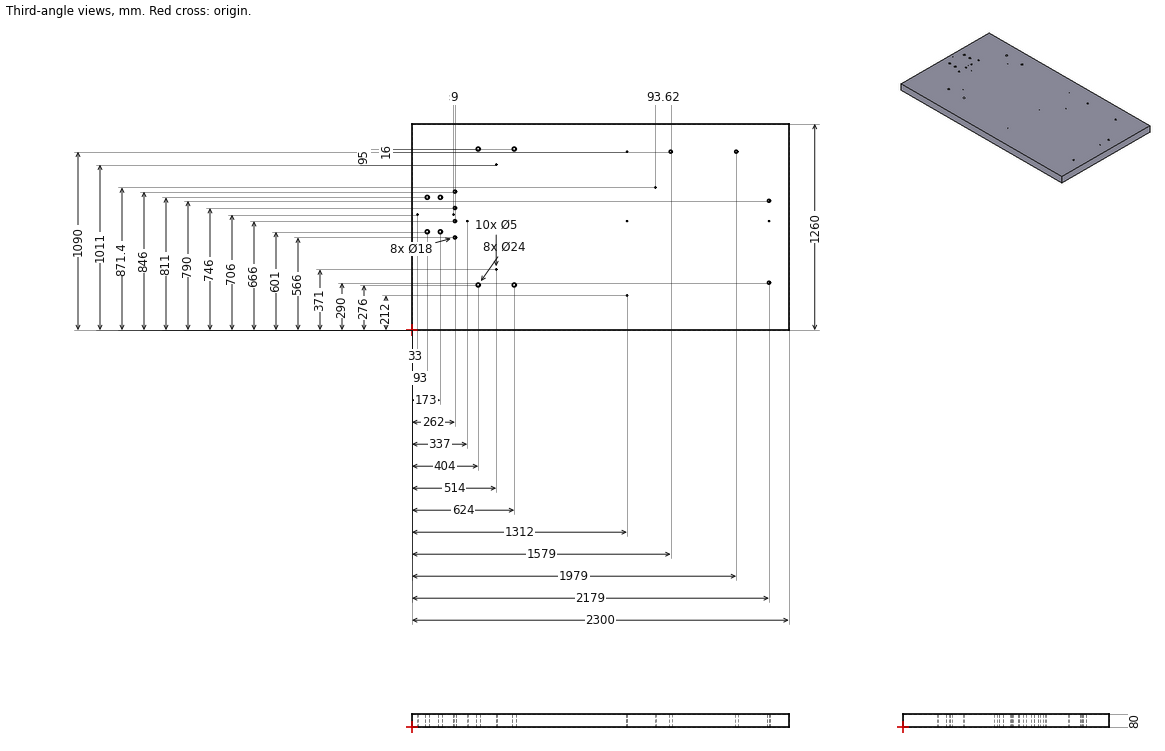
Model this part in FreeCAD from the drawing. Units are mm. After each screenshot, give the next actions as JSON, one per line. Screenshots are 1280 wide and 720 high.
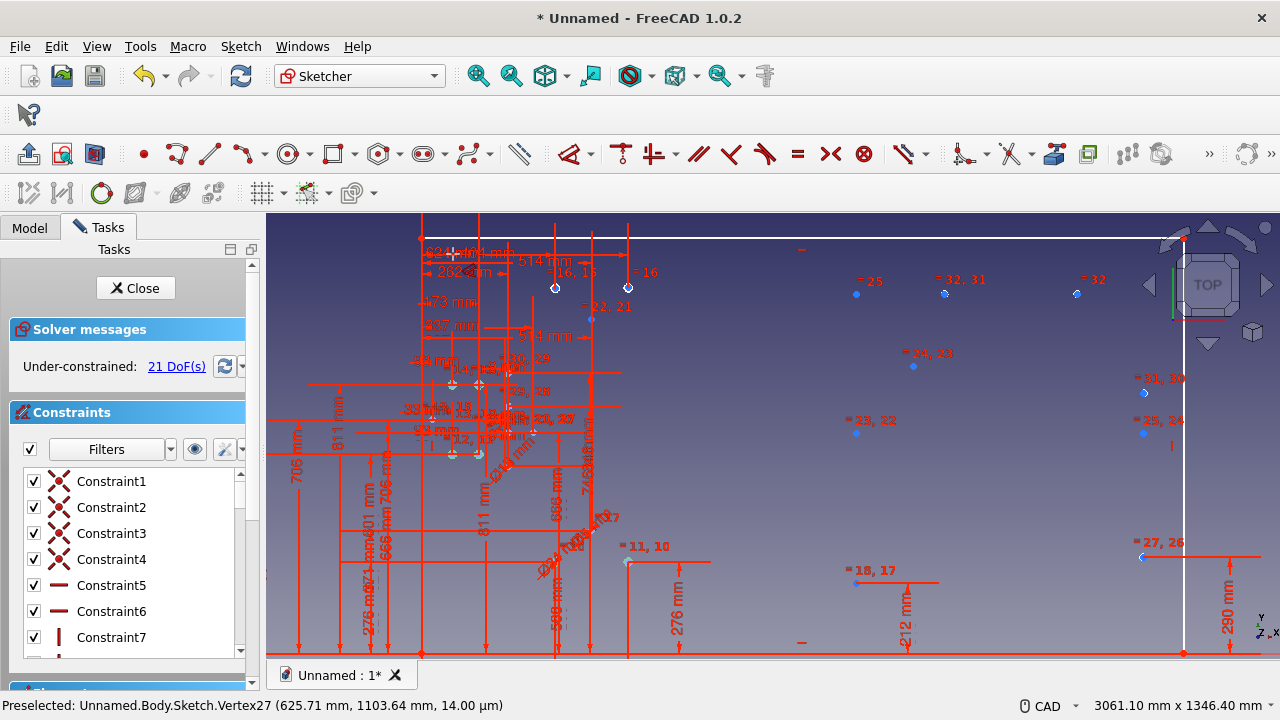
{"action": "left_click", "coordinate": [856, 434]}
{"action": "left_click", "coordinate": [890, 532]}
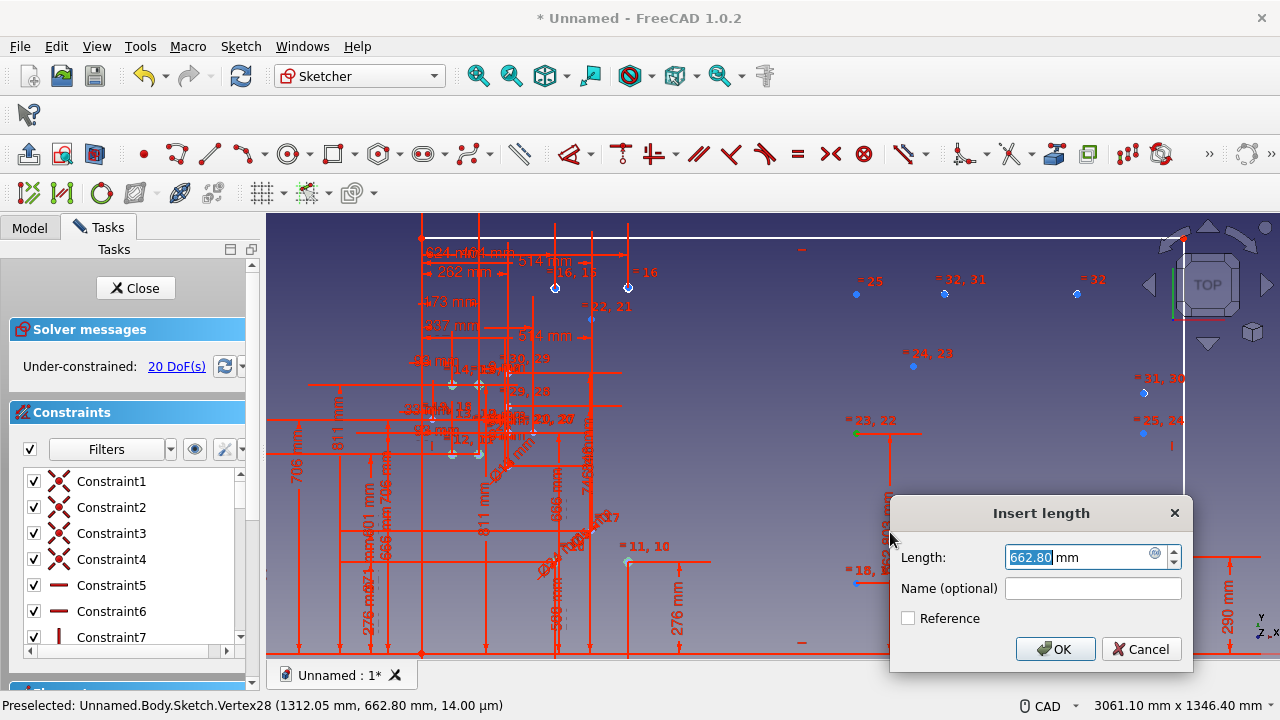
{"action": "type", "text": "666"}
{"action": "key", "text": "Return"}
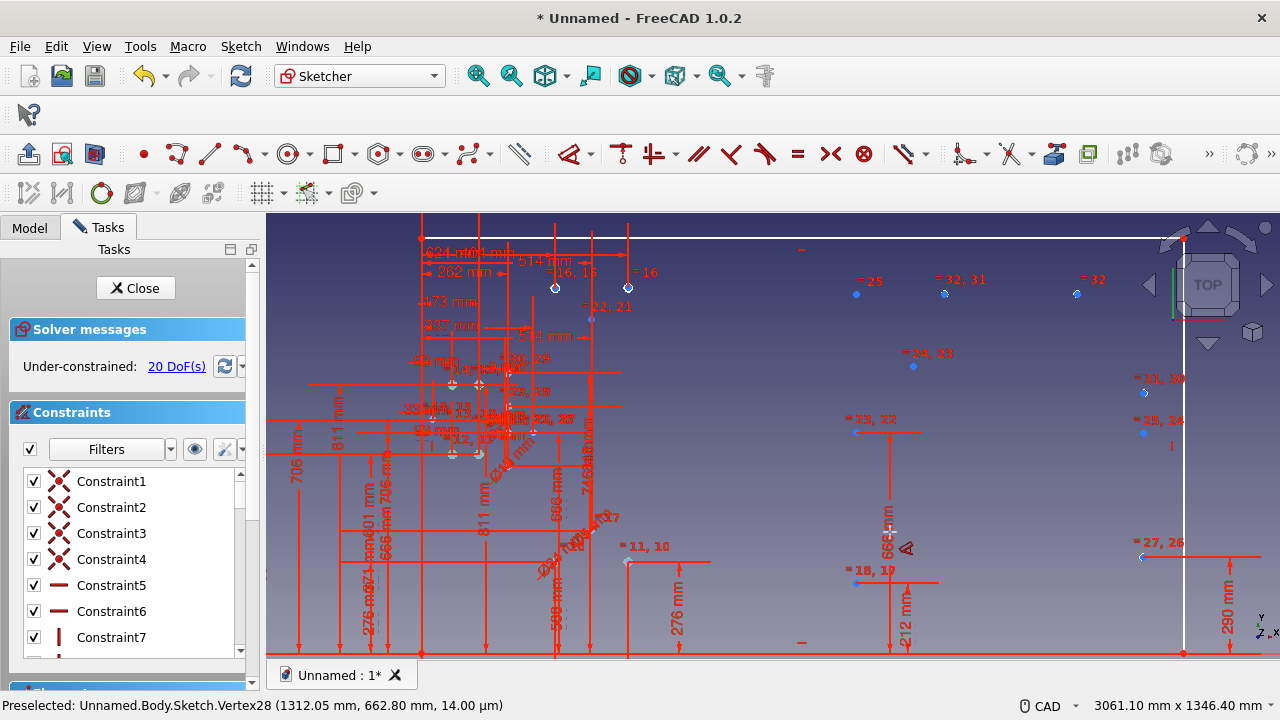
{"action": "scroll", "coordinate": [505, 418], "scroll_direction": "down", "scroll_amount": 2}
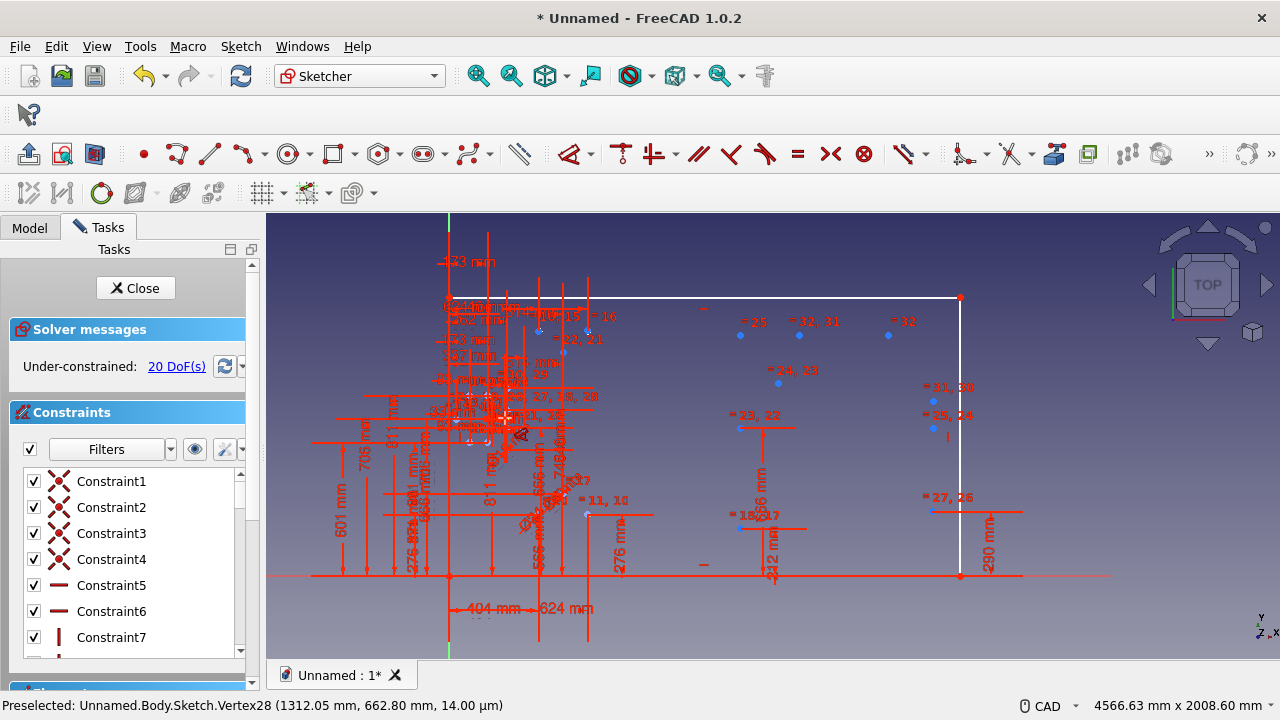
{"action": "left_click", "coordinate": [933, 429]}
{"action": "left_click", "coordinate": [991, 502]}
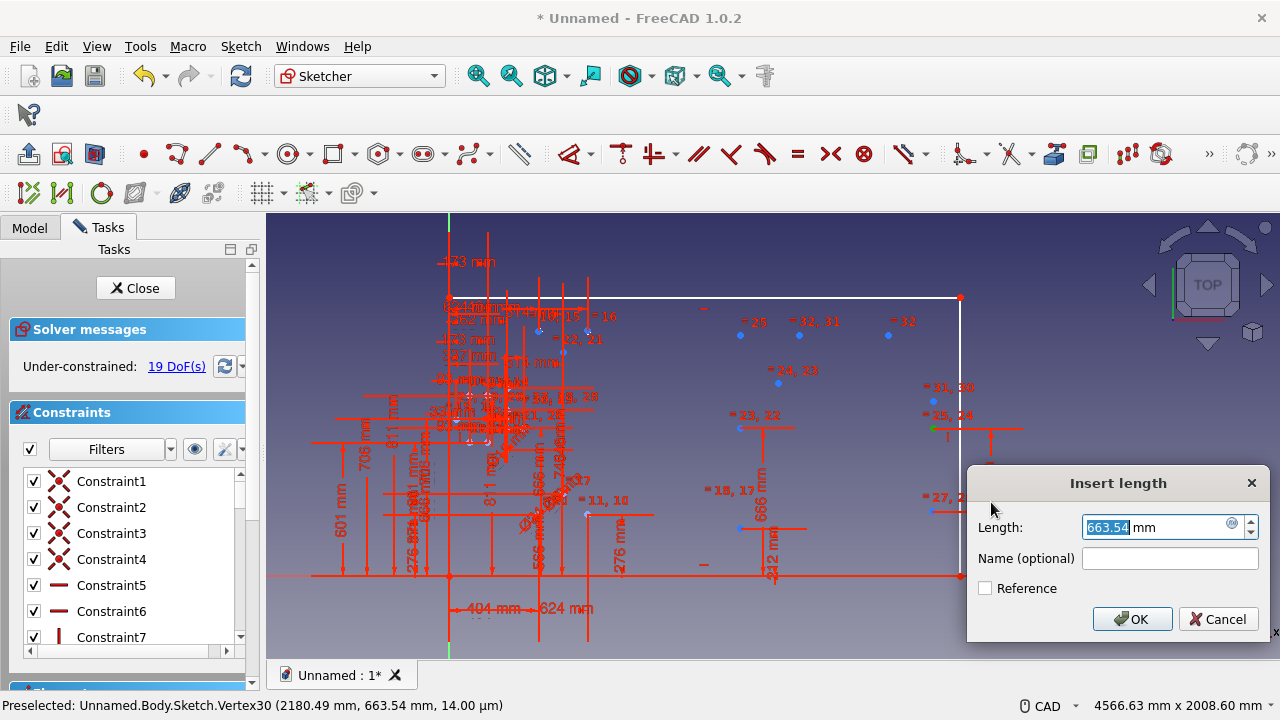
{"action": "type", "text": "666"}
{"action": "key", "text": "Return"}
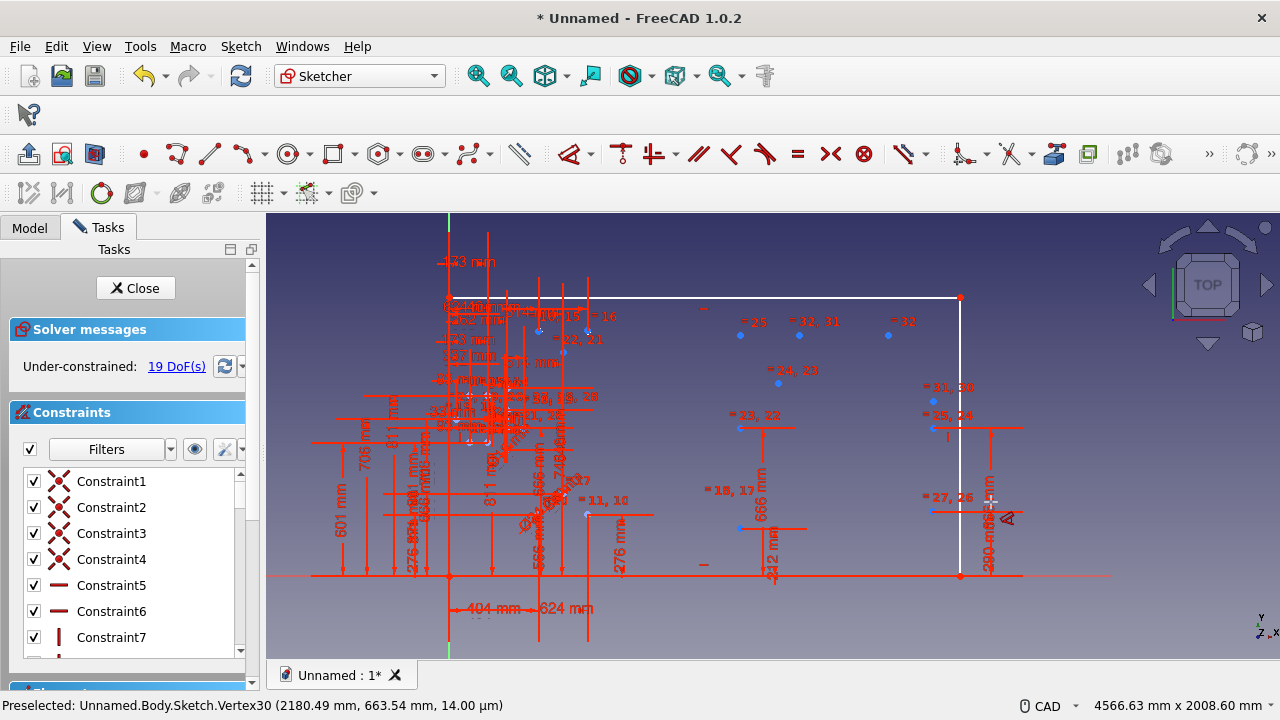
{"action": "left_click", "coordinate": [933, 402]}
{"action": "left_click", "coordinate": [991, 449]}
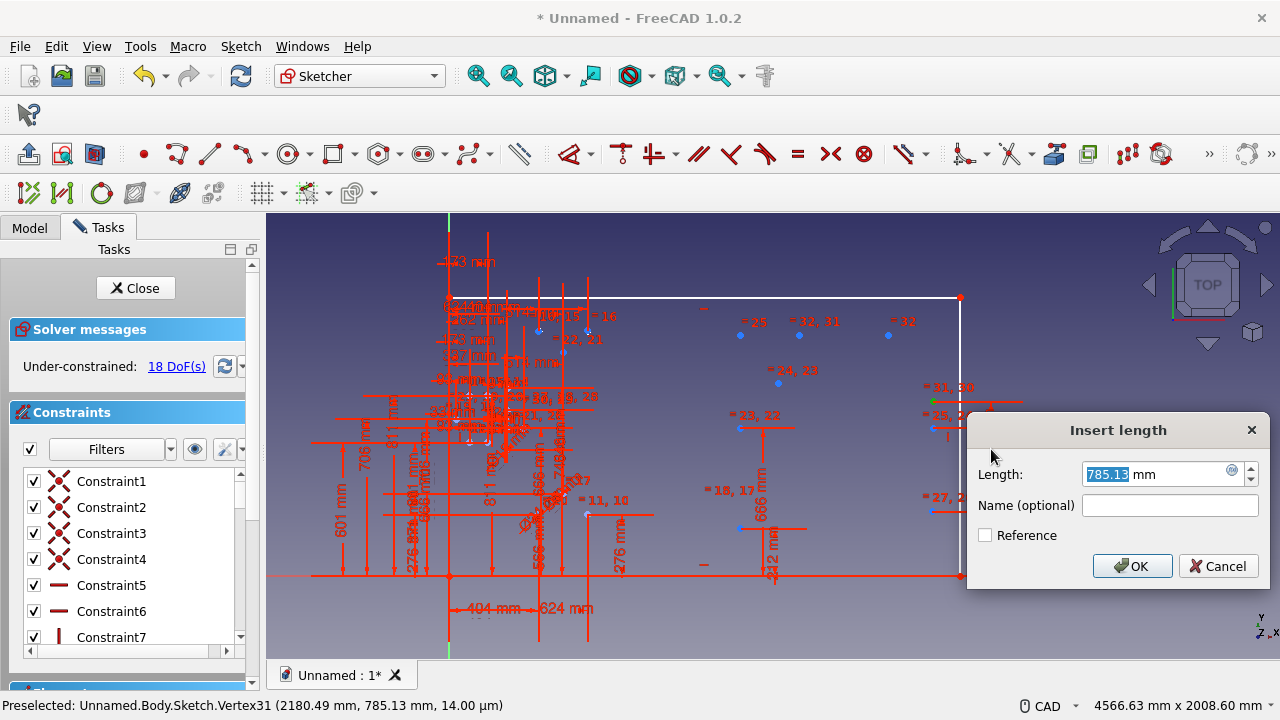
{"action": "type", "text": "790"}
{"action": "key", "text": "Return"}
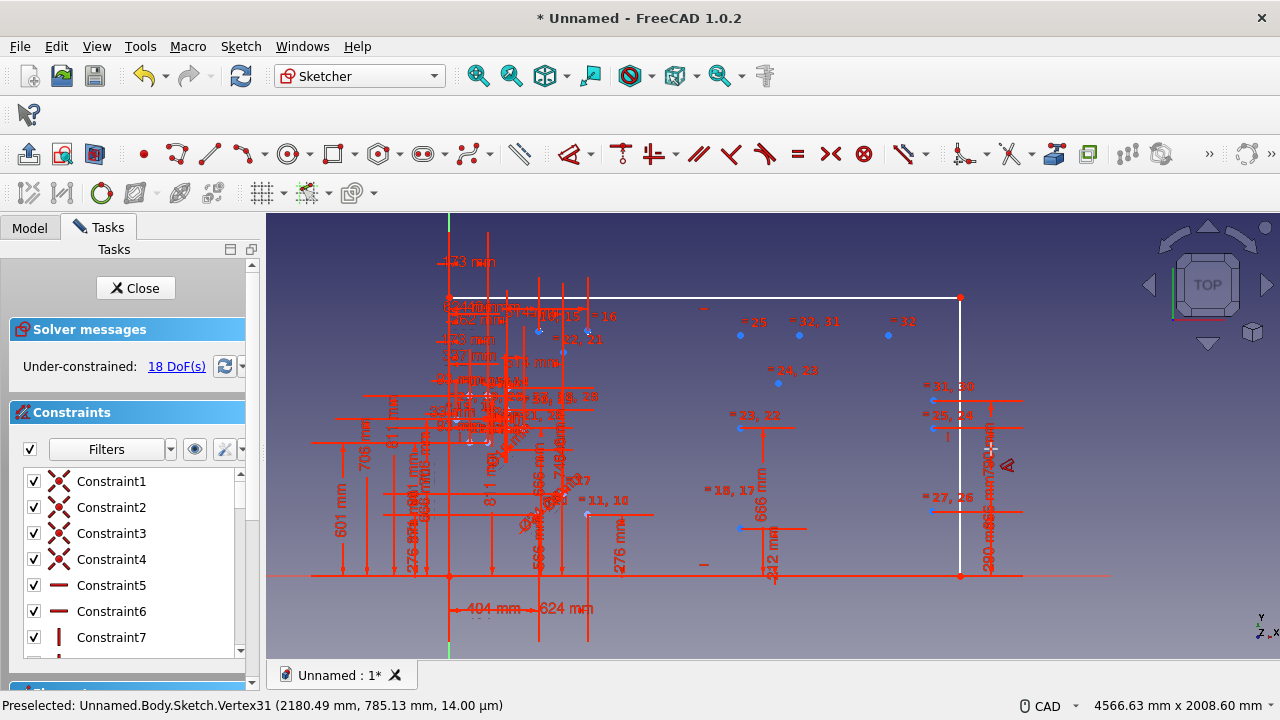
{"action": "scroll", "coordinate": [563, 352], "scroll_direction": "up", "scroll_amount": 4}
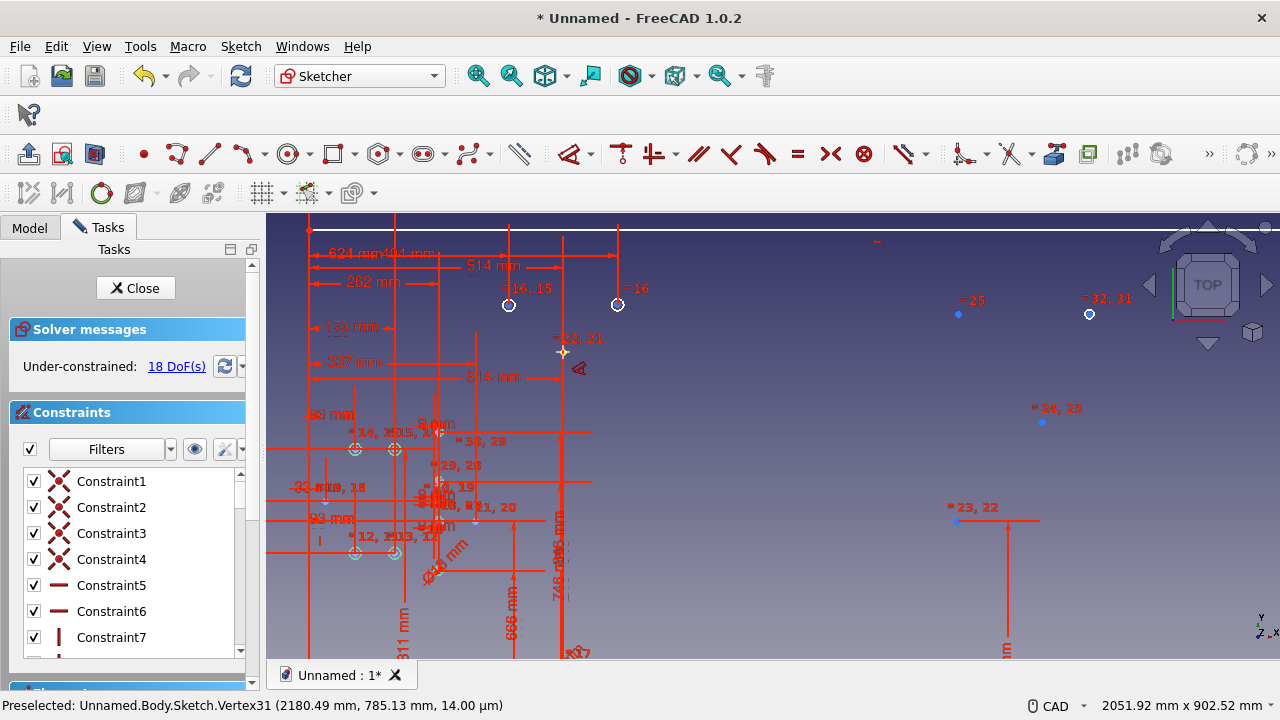
{"action": "left_click", "coordinate": [563, 352]}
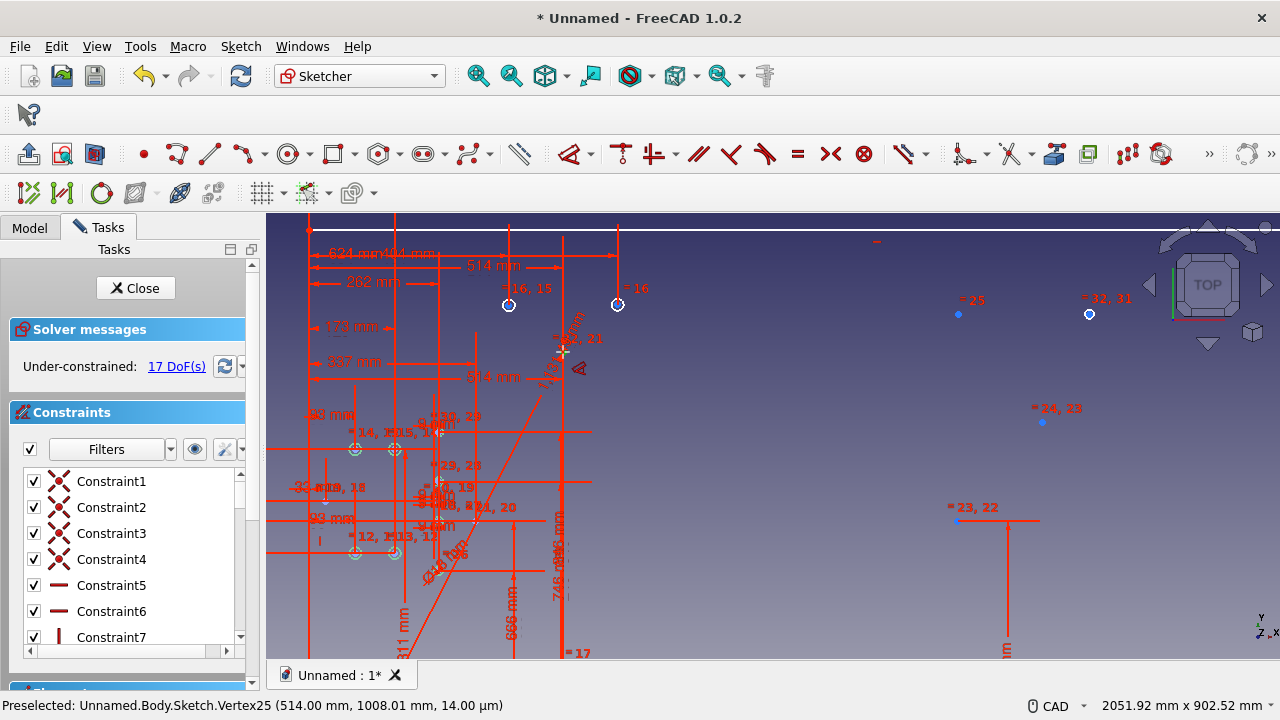
{"action": "left_click", "coordinate": [509, 305]}
{"action": "left_click", "coordinate": [475, 329]}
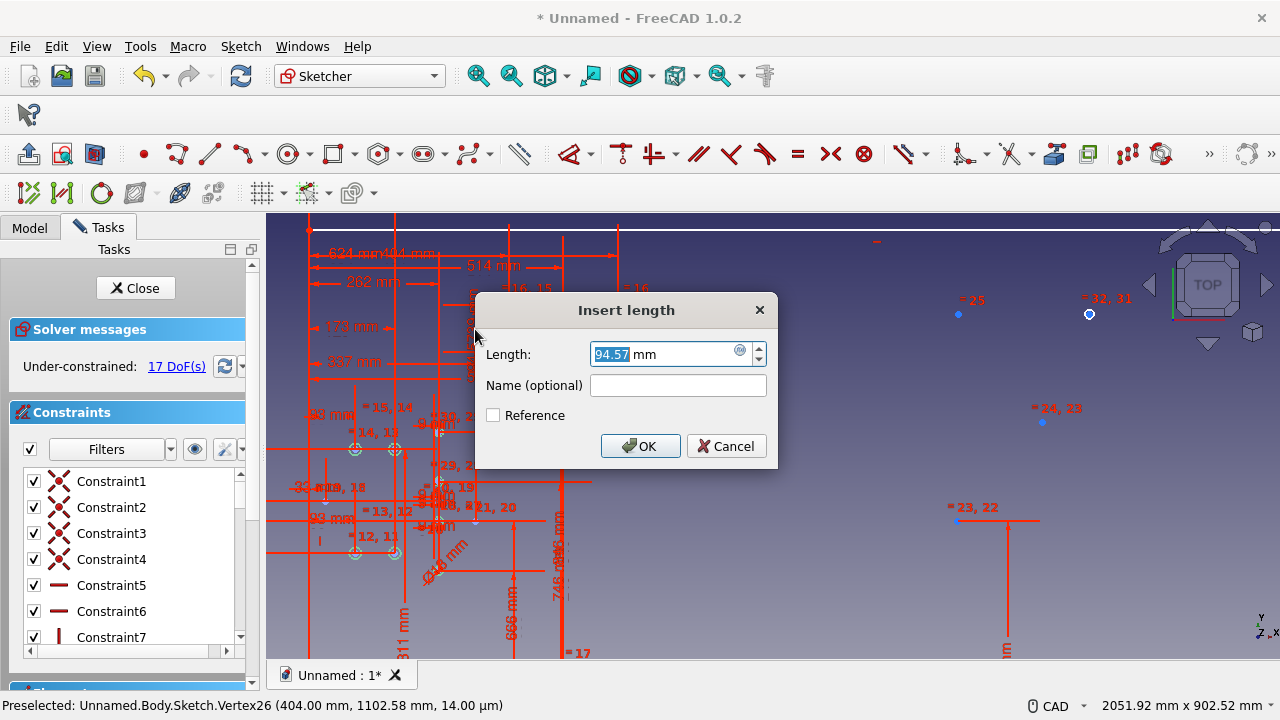
{"action": "type", "text": "95"}
{"action": "key", "text": "Return"}